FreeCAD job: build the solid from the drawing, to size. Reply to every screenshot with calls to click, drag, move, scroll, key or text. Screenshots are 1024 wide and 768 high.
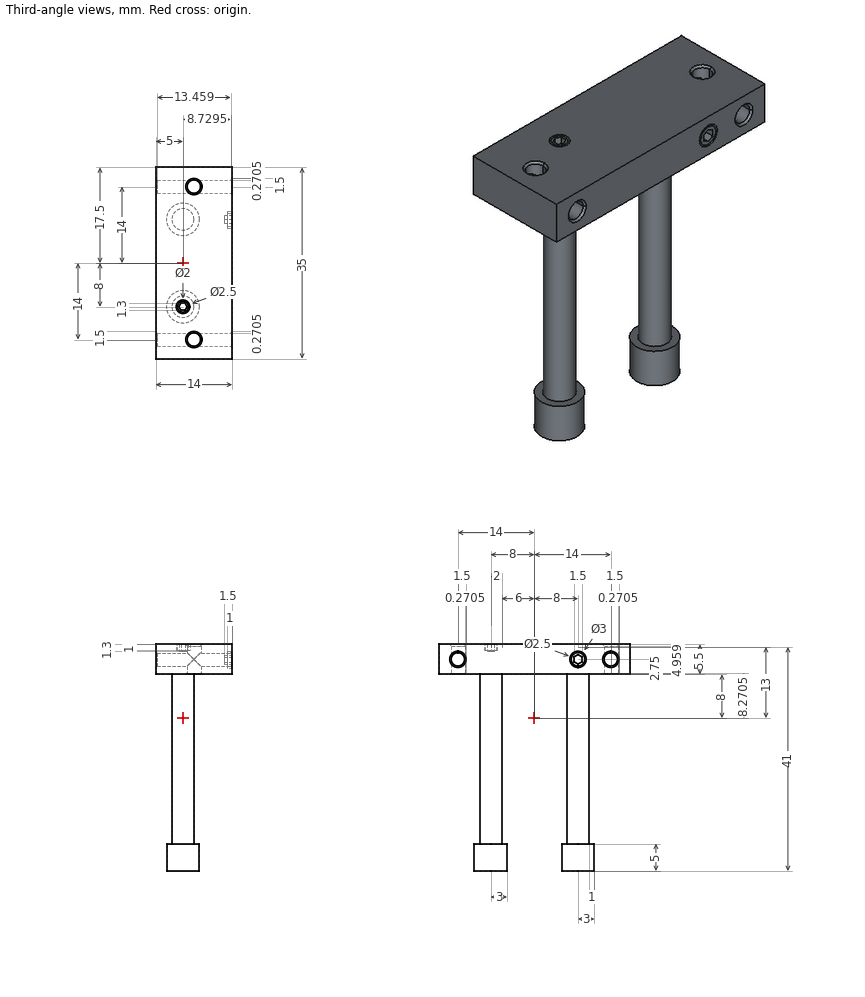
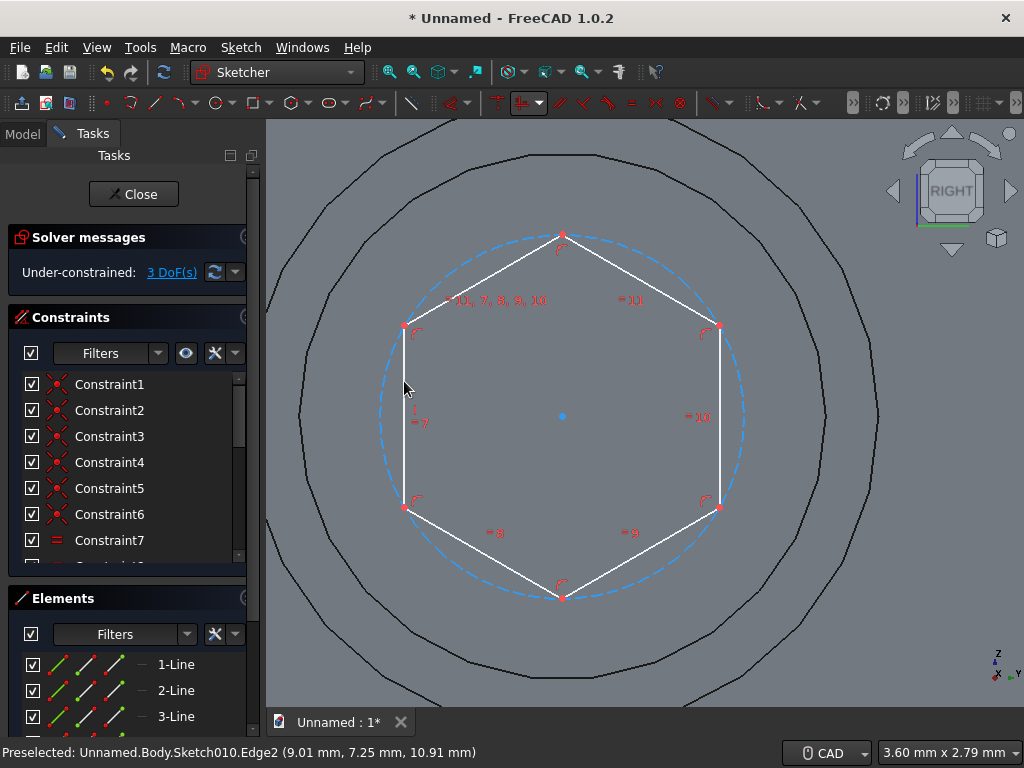
click(450, 104)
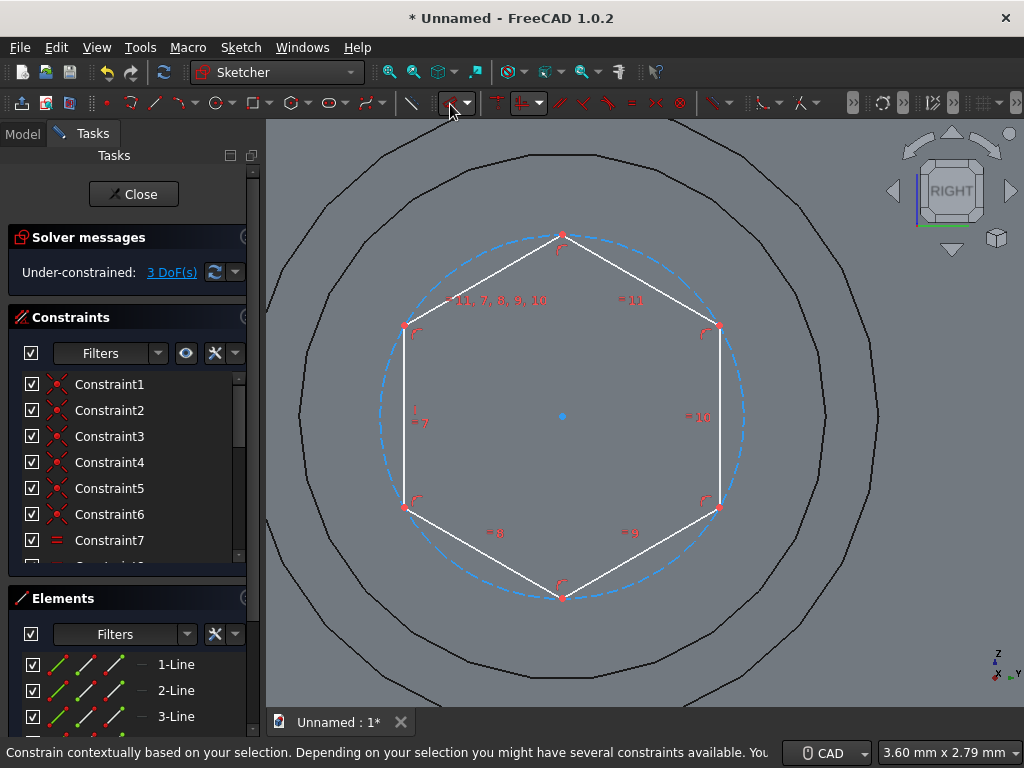
click(562, 417)
click(428, 383)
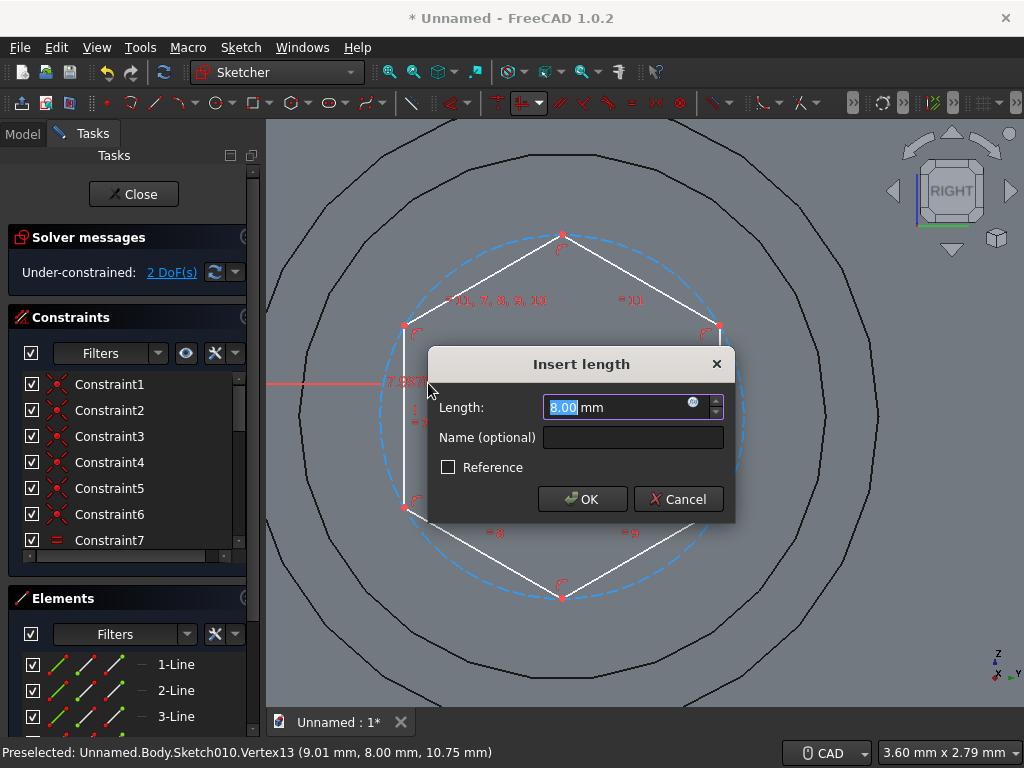
text(8)
key(Return)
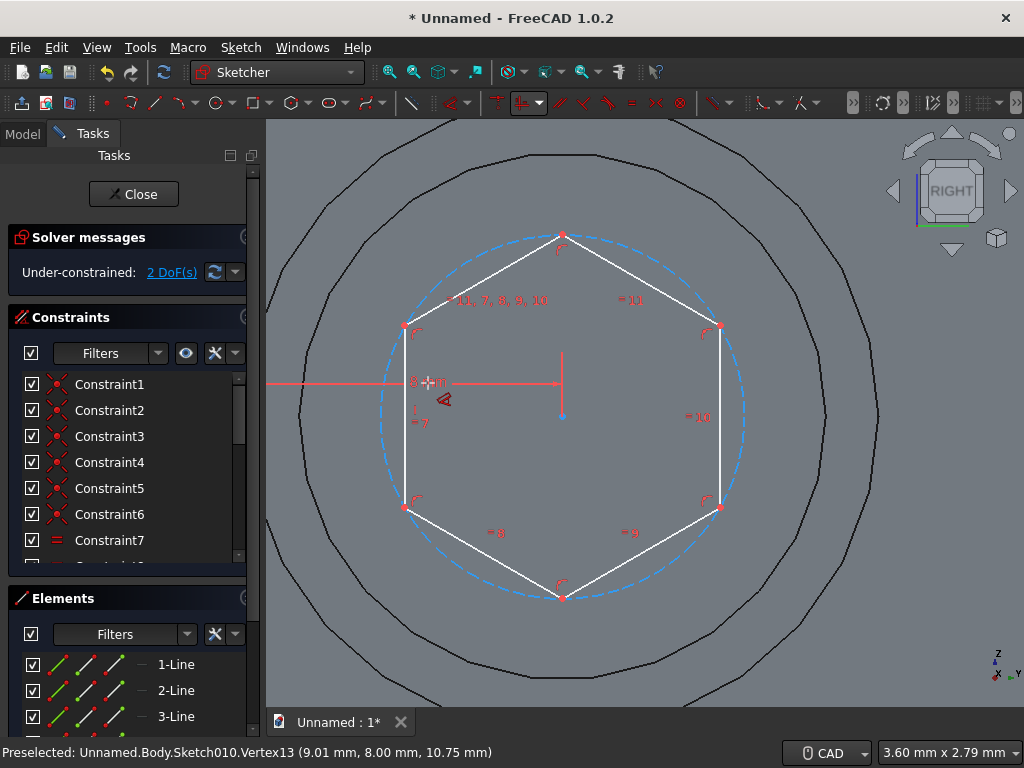
click(405, 326)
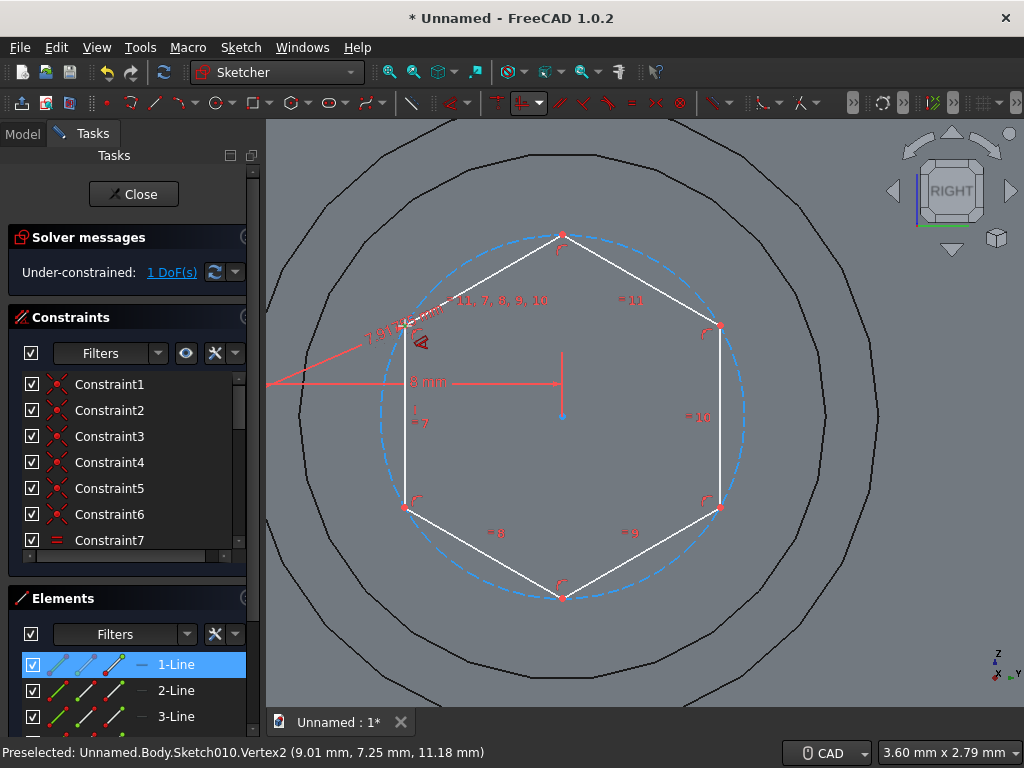
click(720, 508)
click(562, 542)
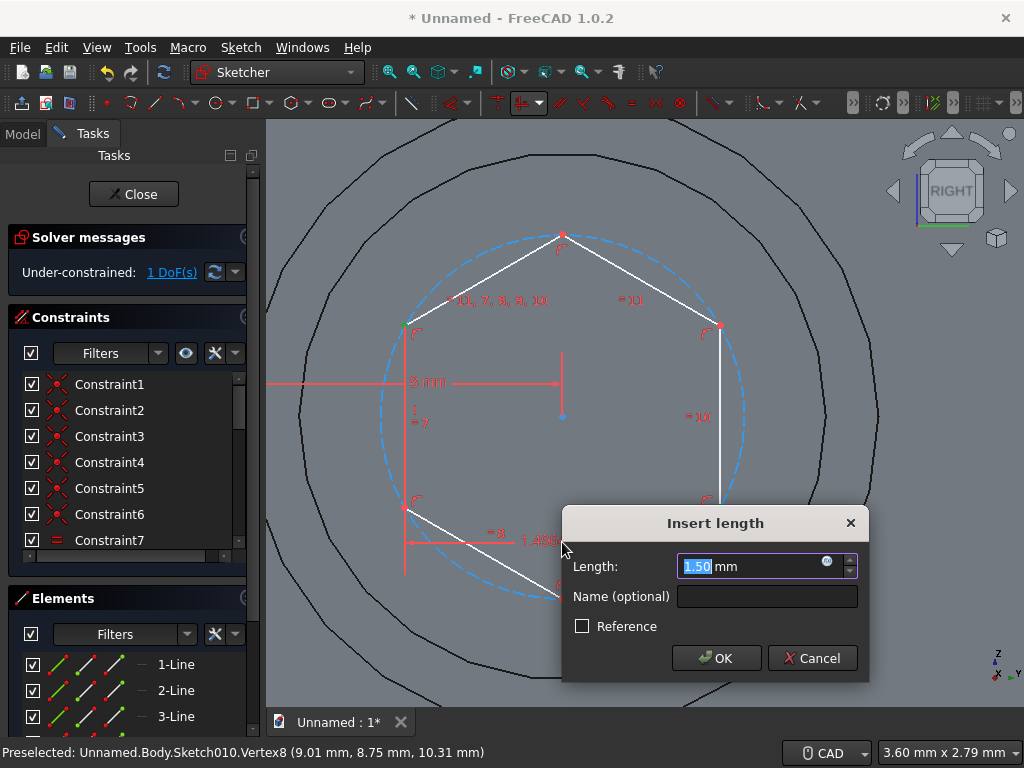
text(1.5)
key(Return)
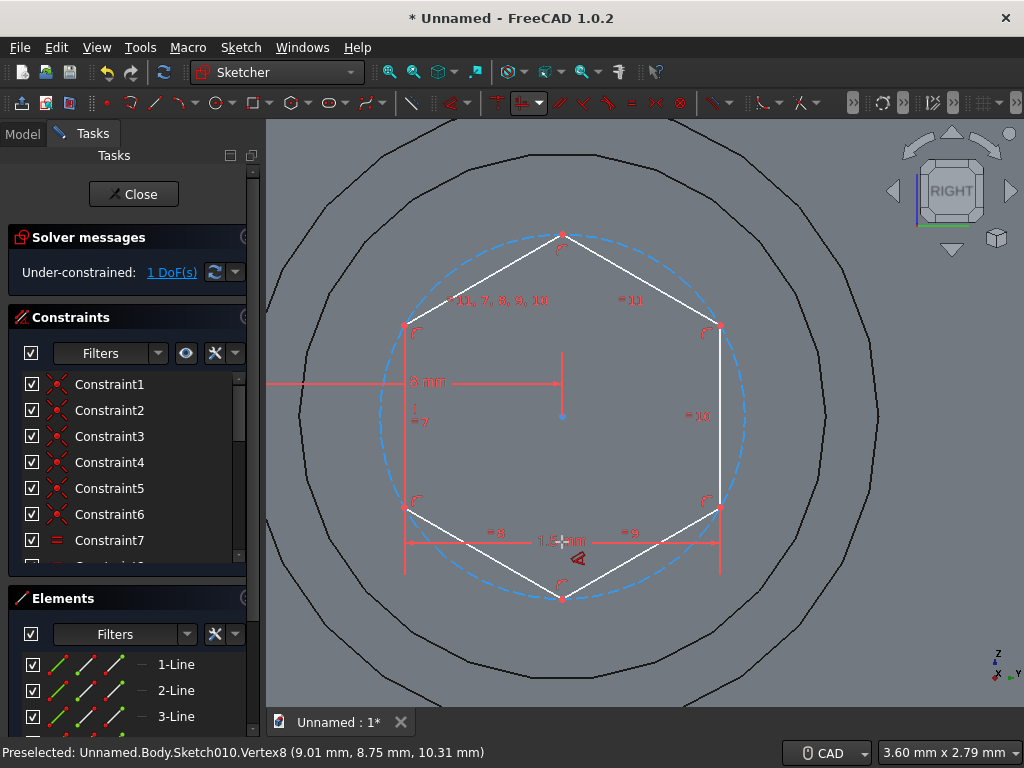
click(562, 417)
click(596, 488)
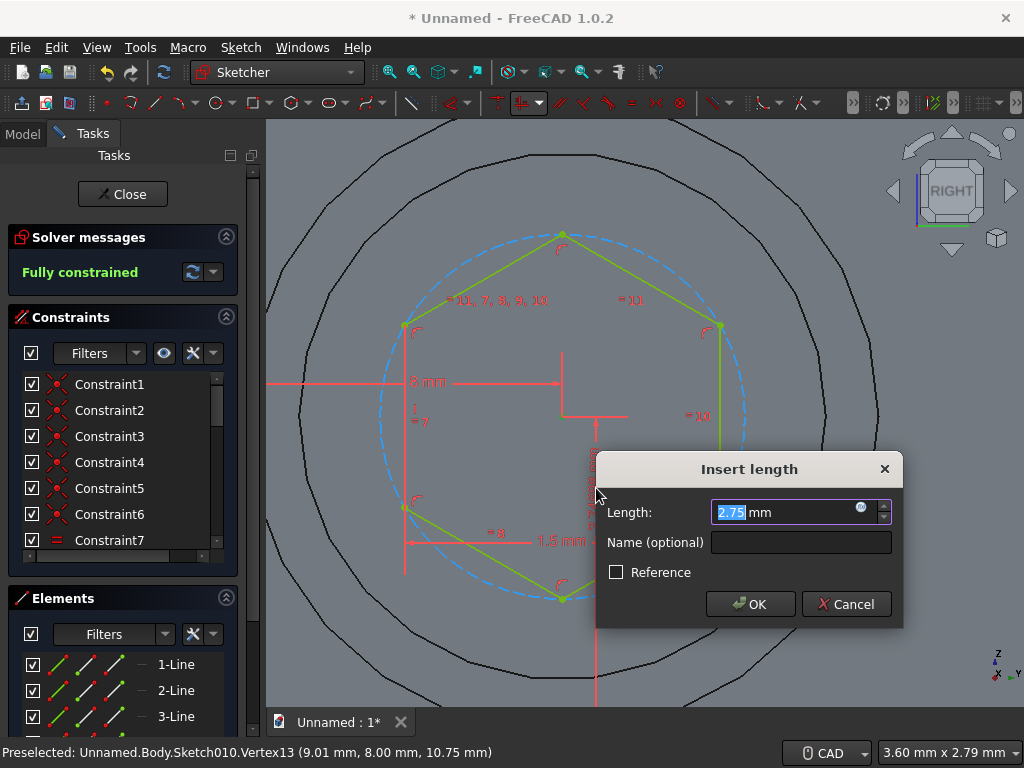
text(2.75)
key(Return)
key(Escape)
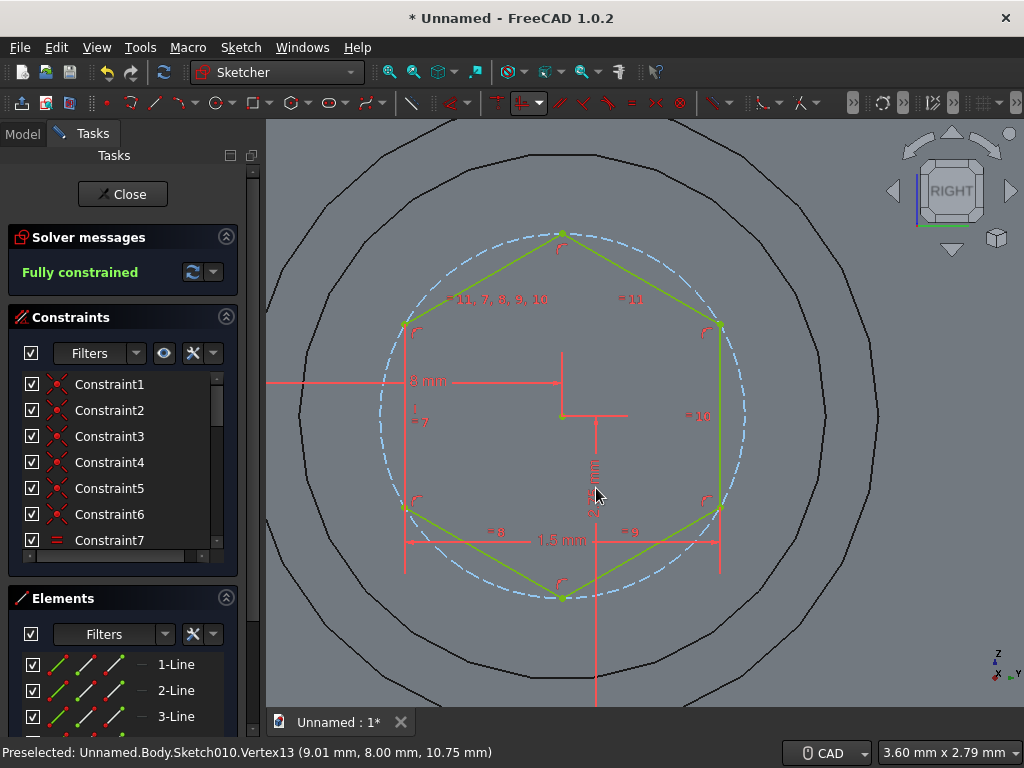
click(123, 194)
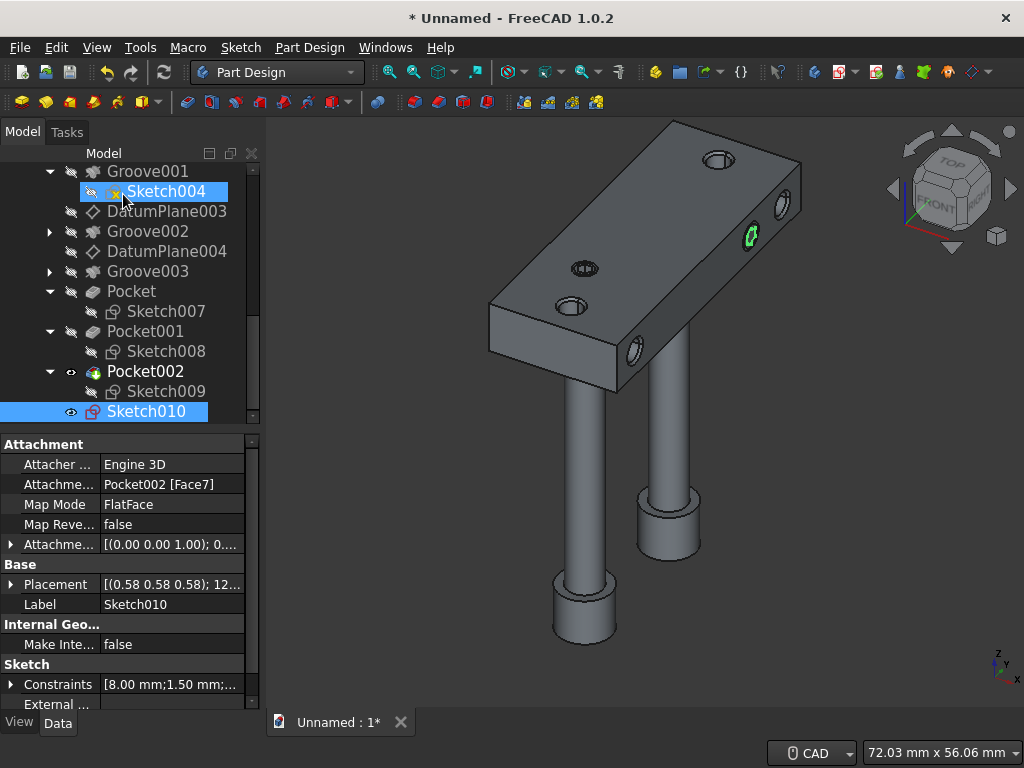
click(188, 102)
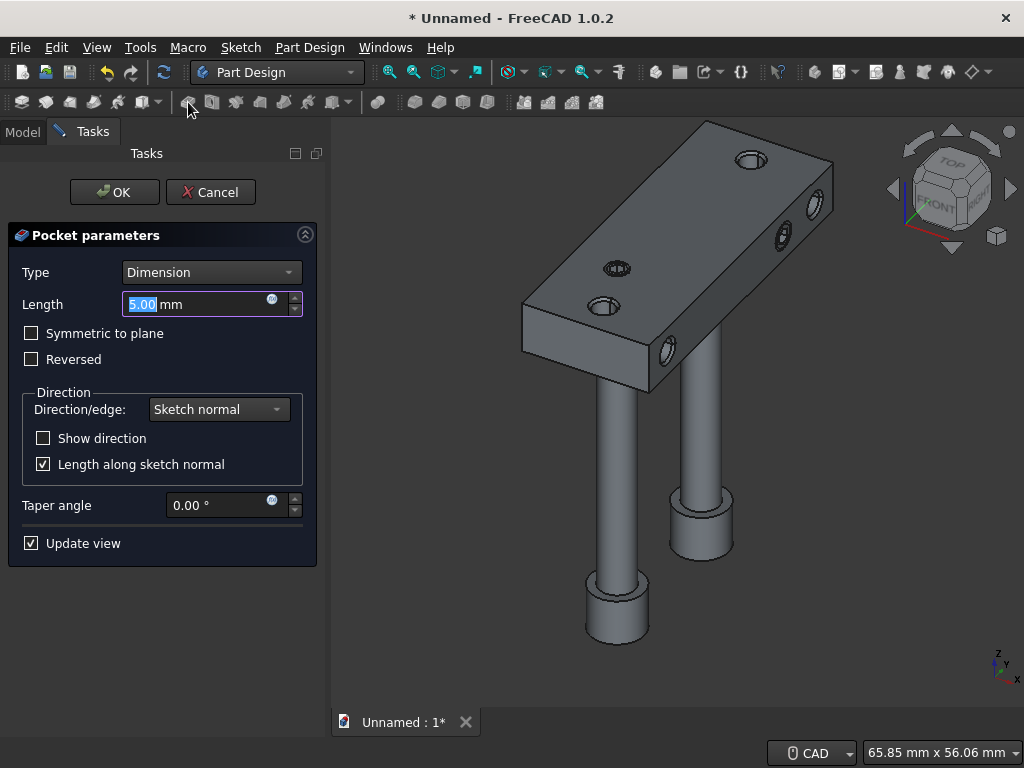
text(1.5)
key(Tab)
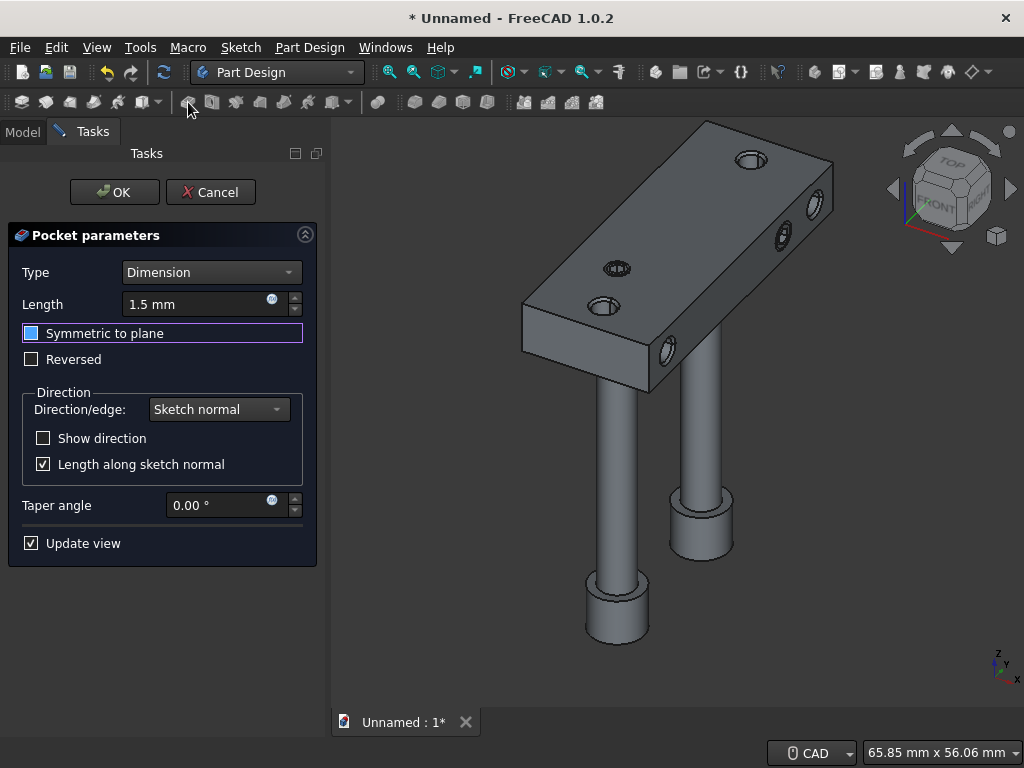
click(115, 192)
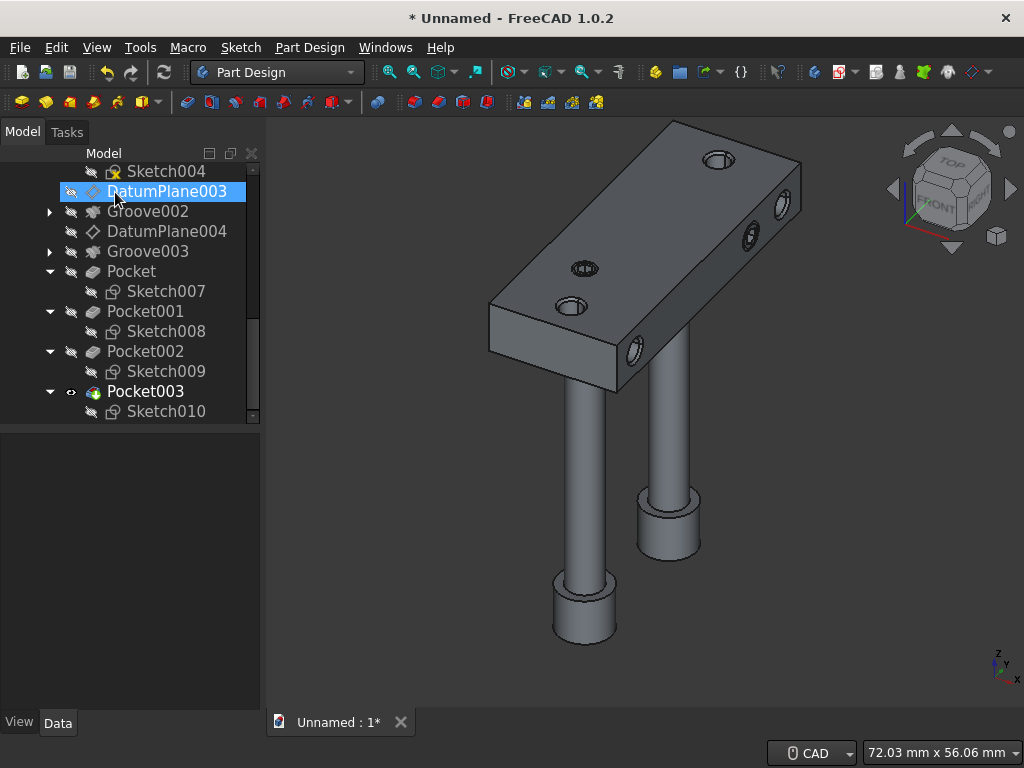
key(0)